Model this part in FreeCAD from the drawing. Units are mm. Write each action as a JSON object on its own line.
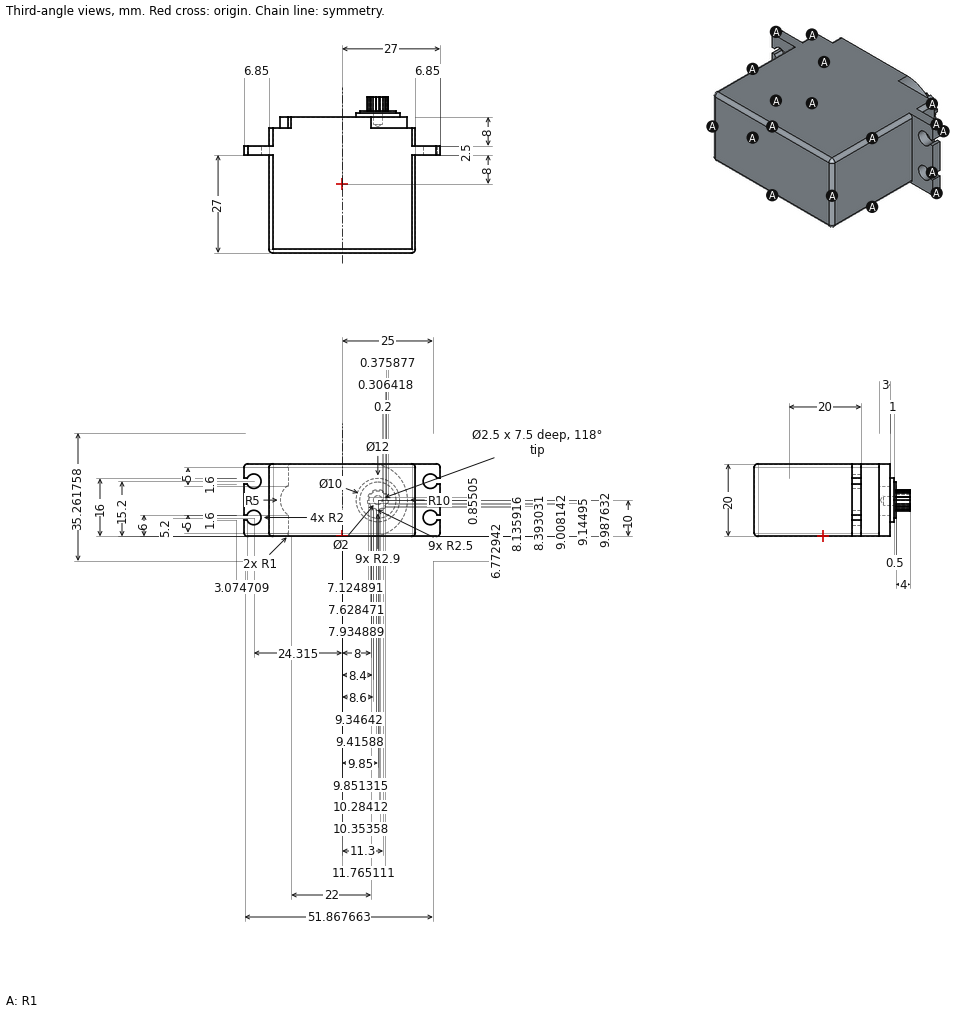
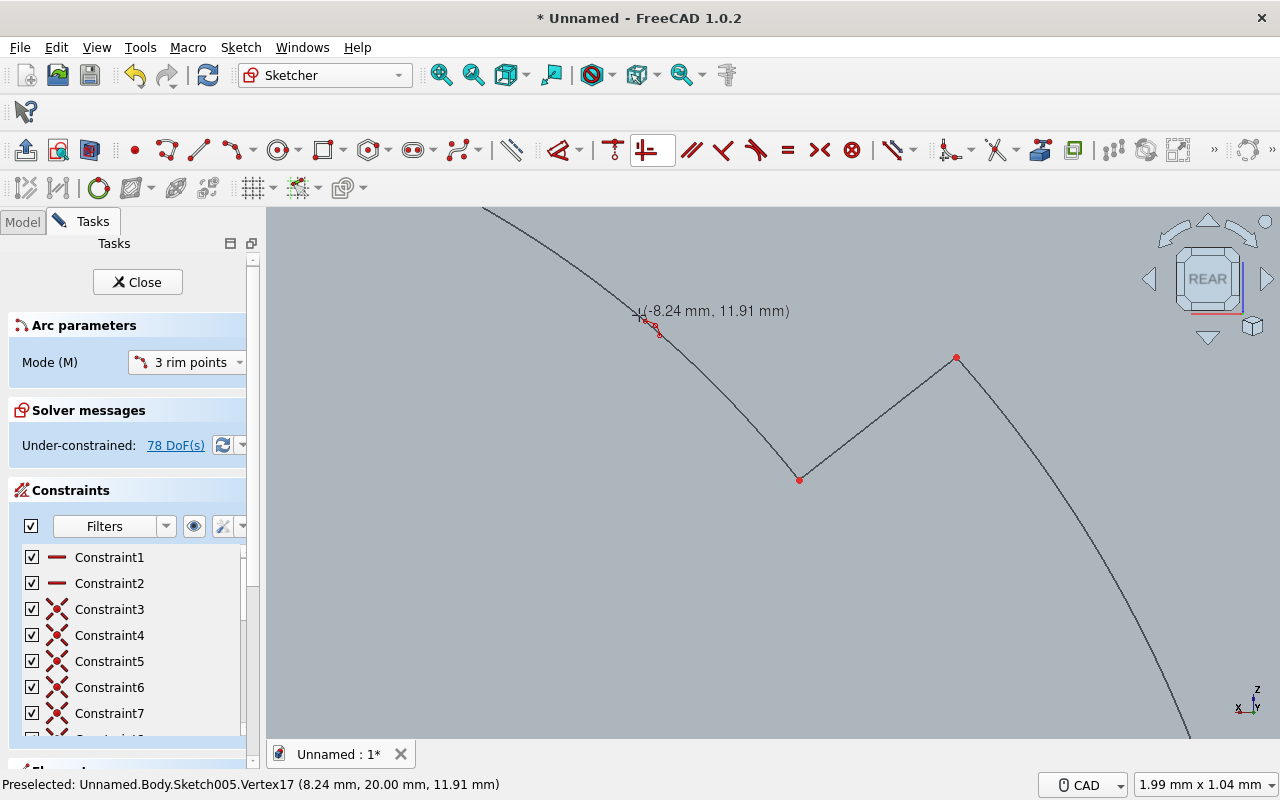
{"action": "scroll", "coordinate": [658, 335], "scroll_direction": "down", "scroll_amount": 15}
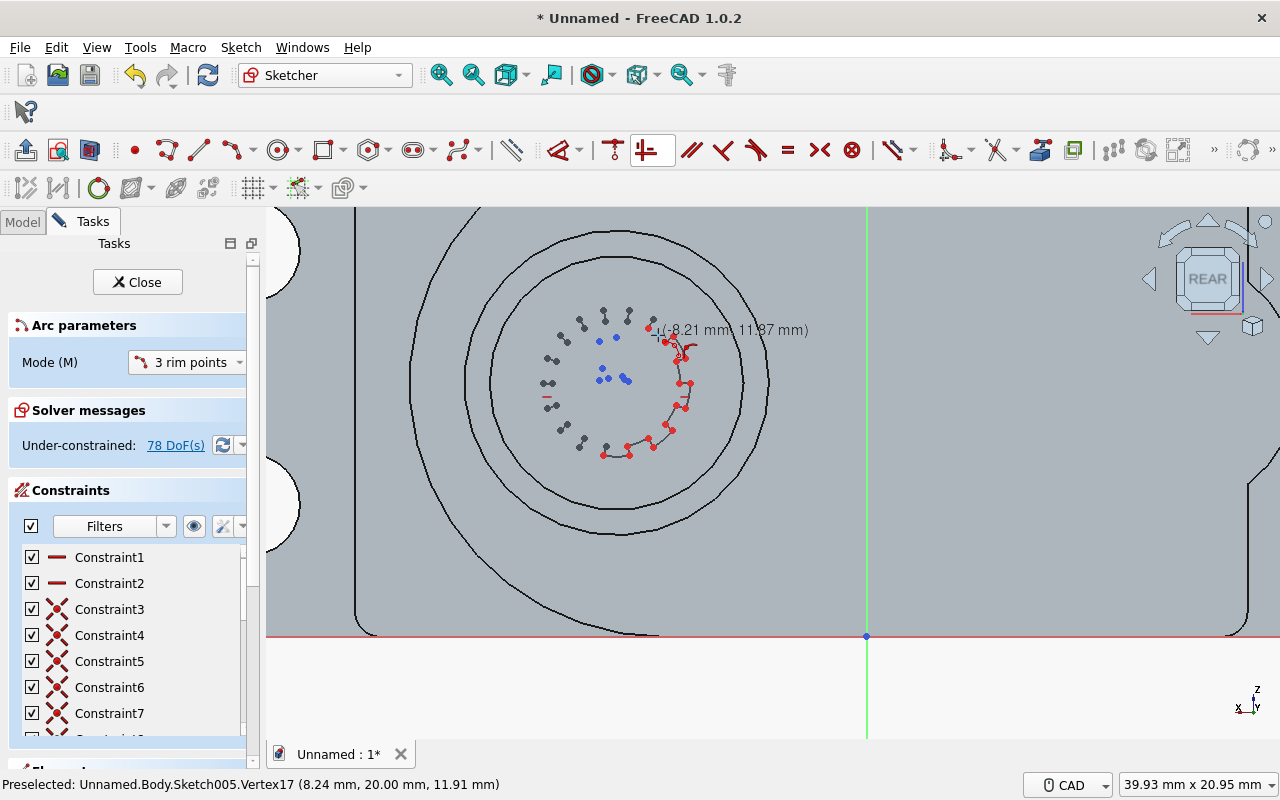
{"action": "scroll", "coordinate": [653, 319], "scroll_direction": "up", "scroll_amount": 6}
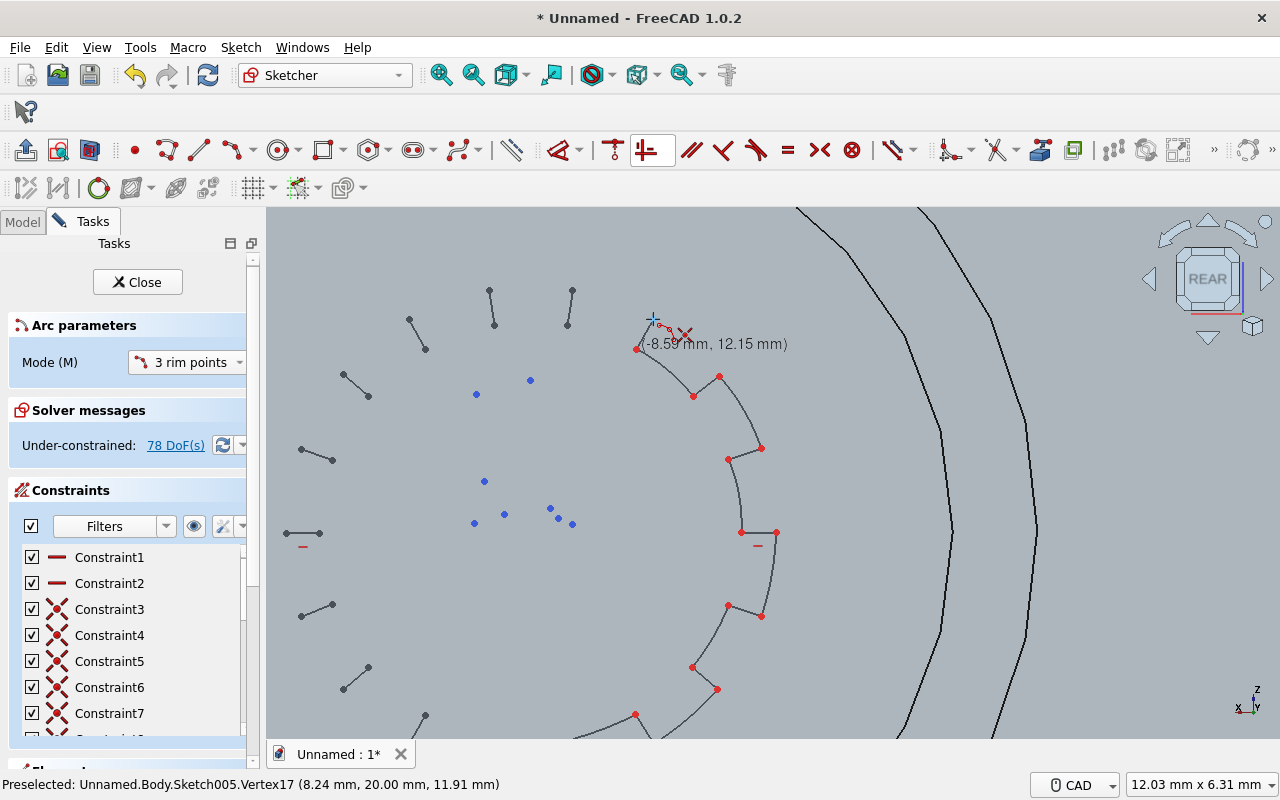
{"action": "left_click", "coordinate": [653, 320]}
{"action": "left_click", "coordinate": [573, 291]}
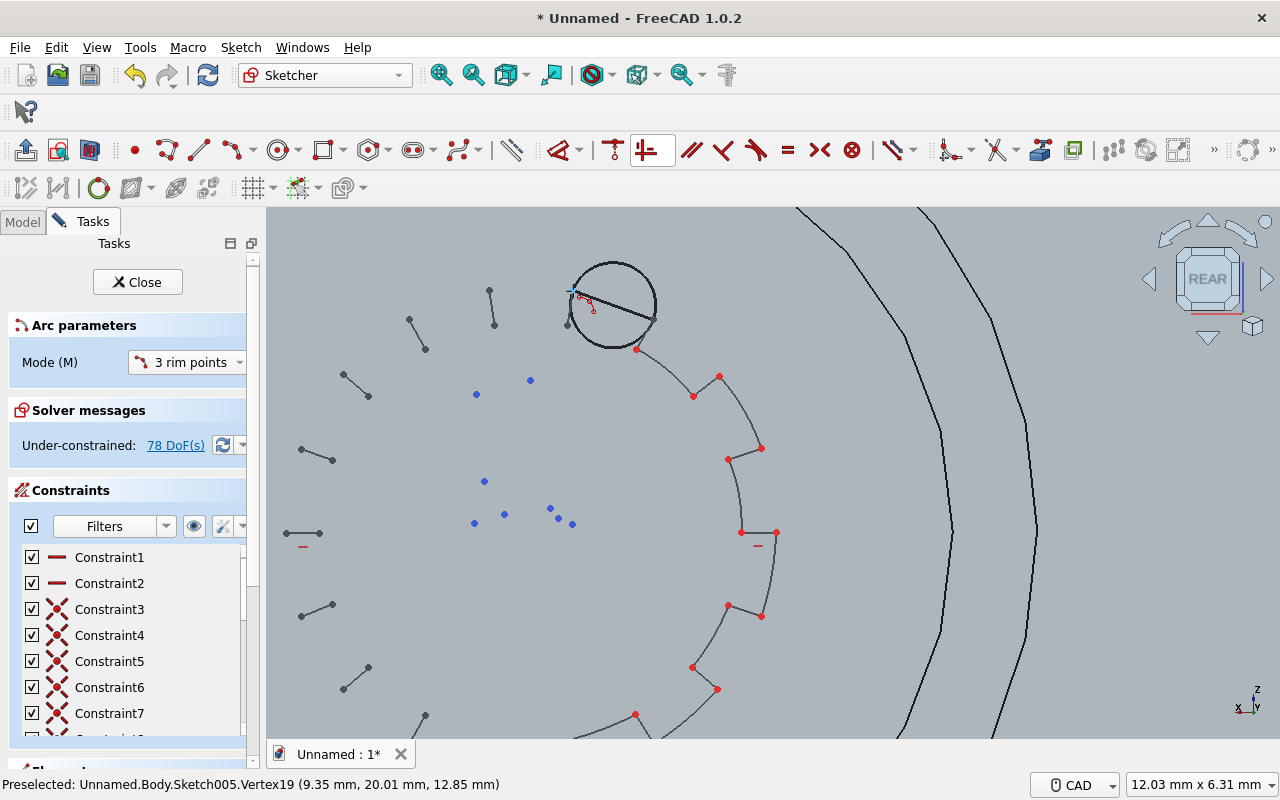
{"action": "scroll", "coordinate": [615, 301], "scroll_direction": "up", "scroll_amount": 8}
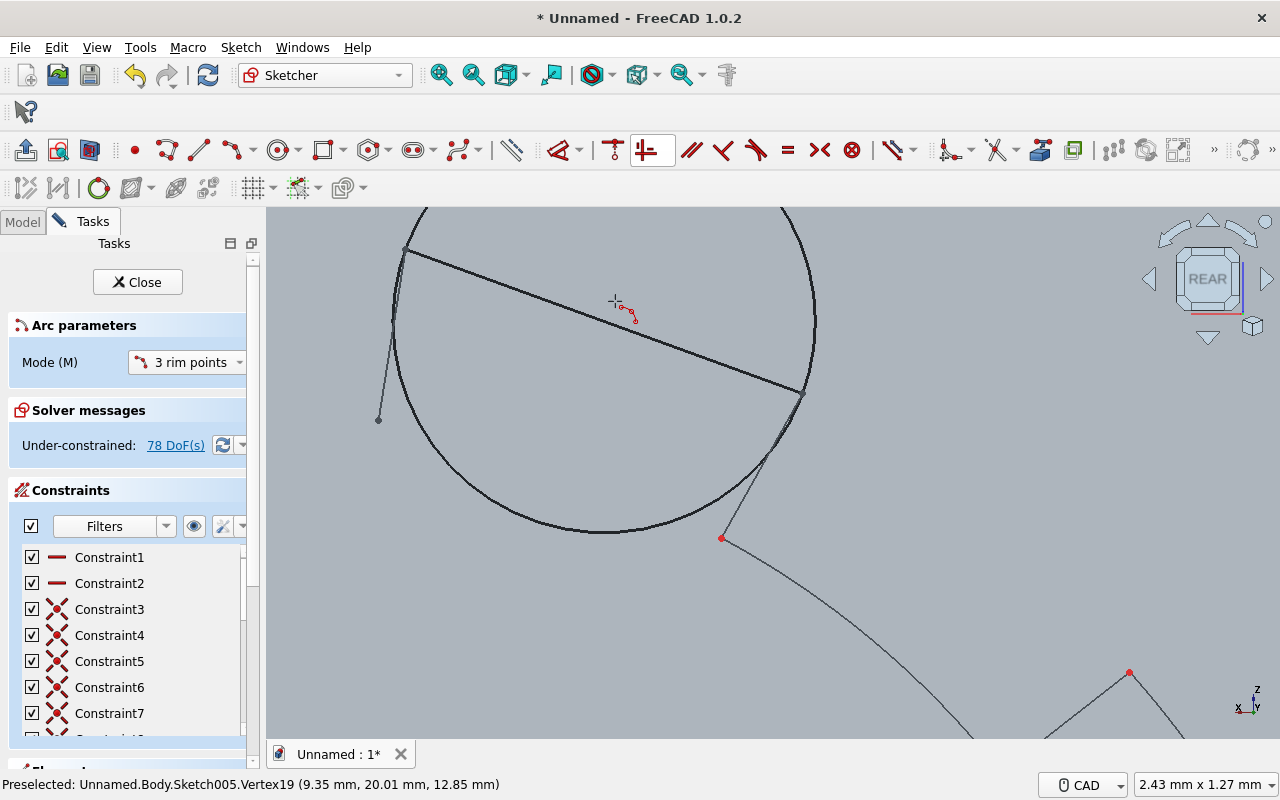
{"action": "left_click", "coordinate": [613, 299]}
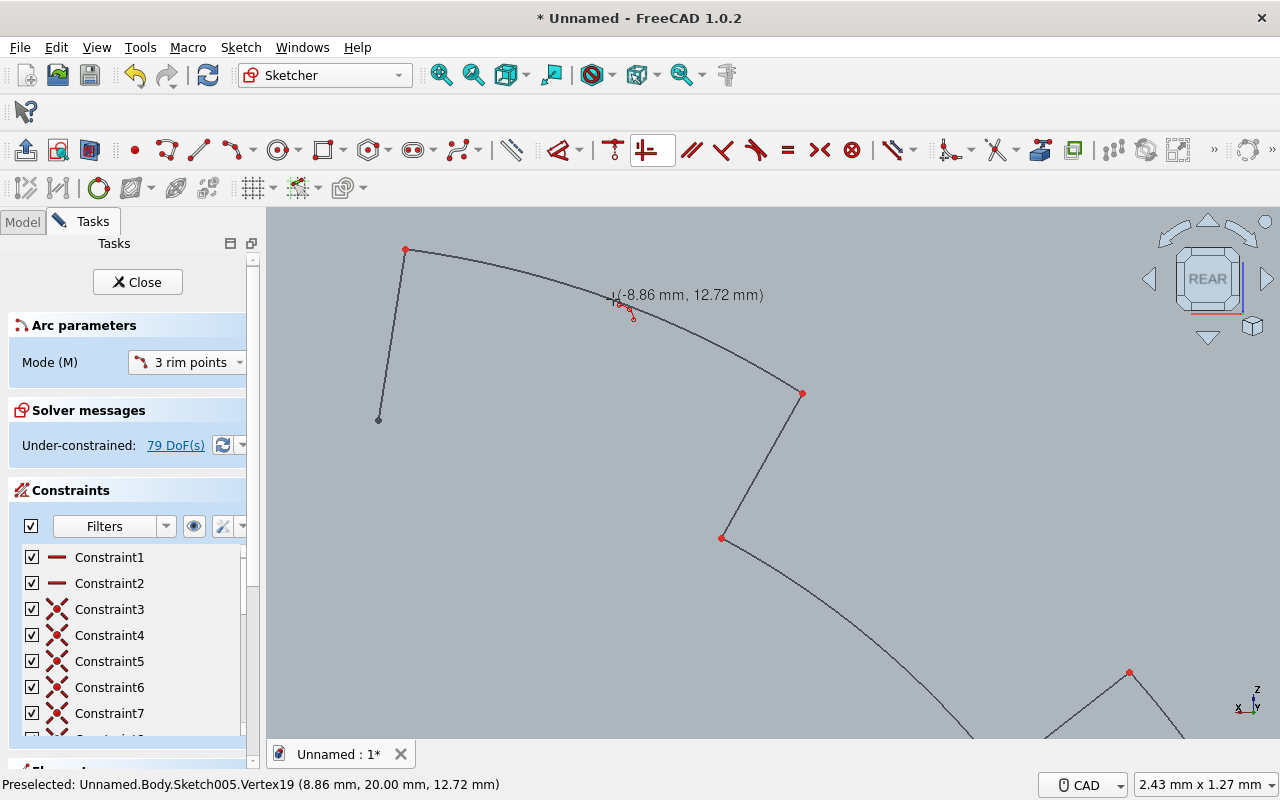
{"action": "scroll", "coordinate": [643, 314], "scroll_direction": "down", "scroll_amount": 14}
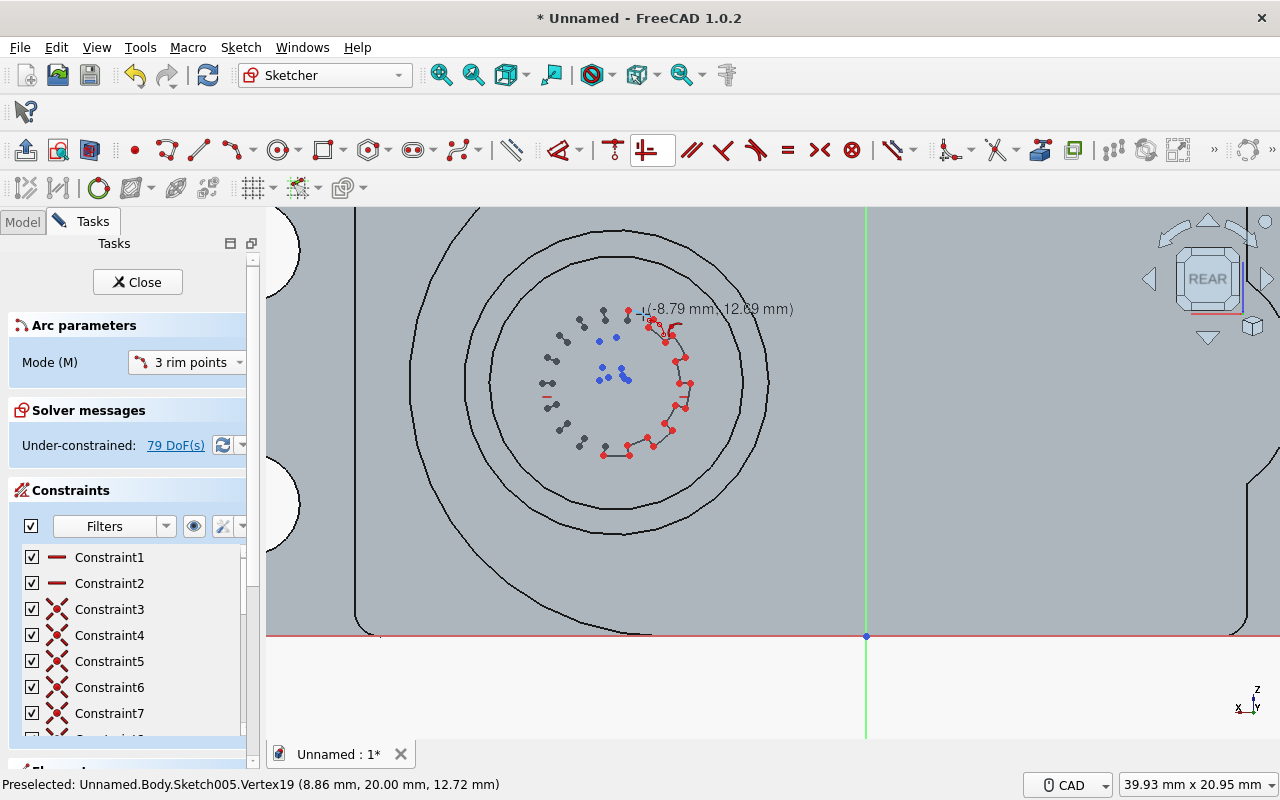
{"action": "scroll", "coordinate": [627, 320], "scroll_direction": "up", "scroll_amount": 6}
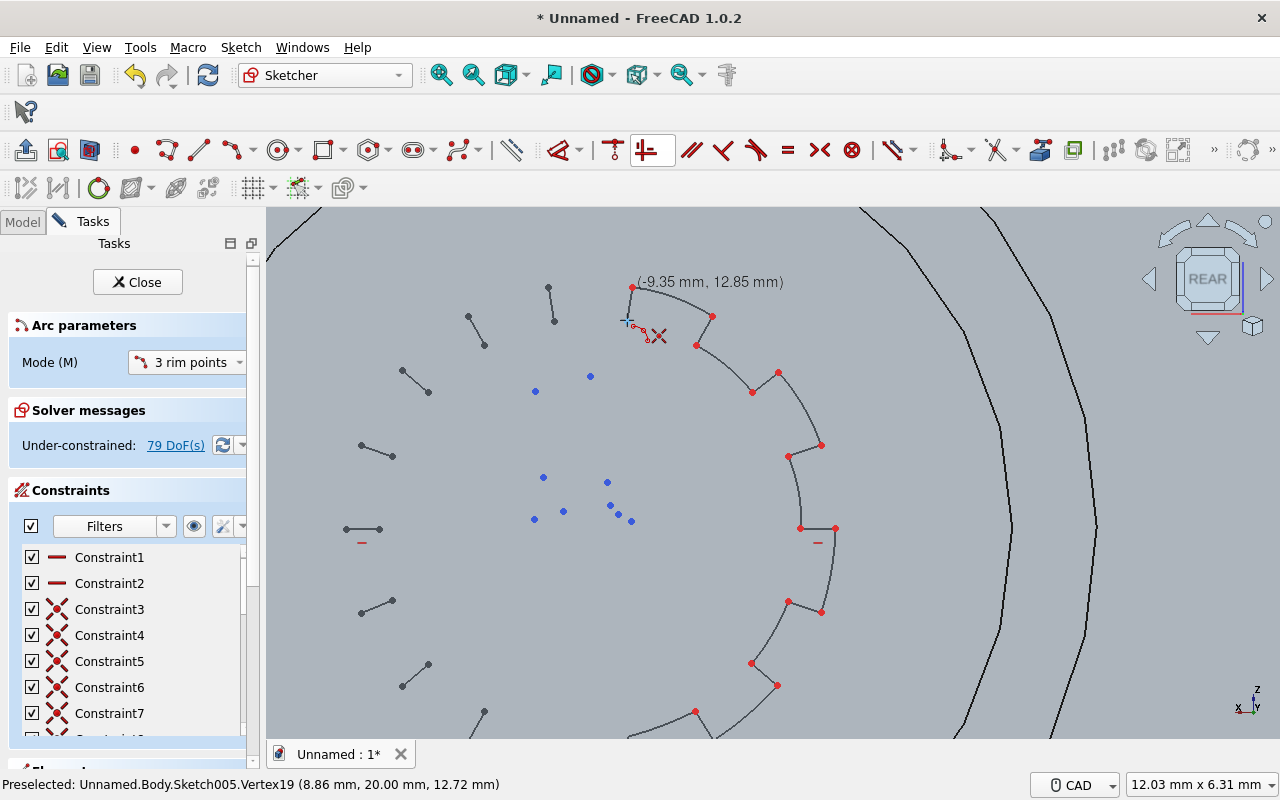
{"action": "left_click", "coordinate": [627, 322]}
{"action": "left_click", "coordinate": [554, 322]}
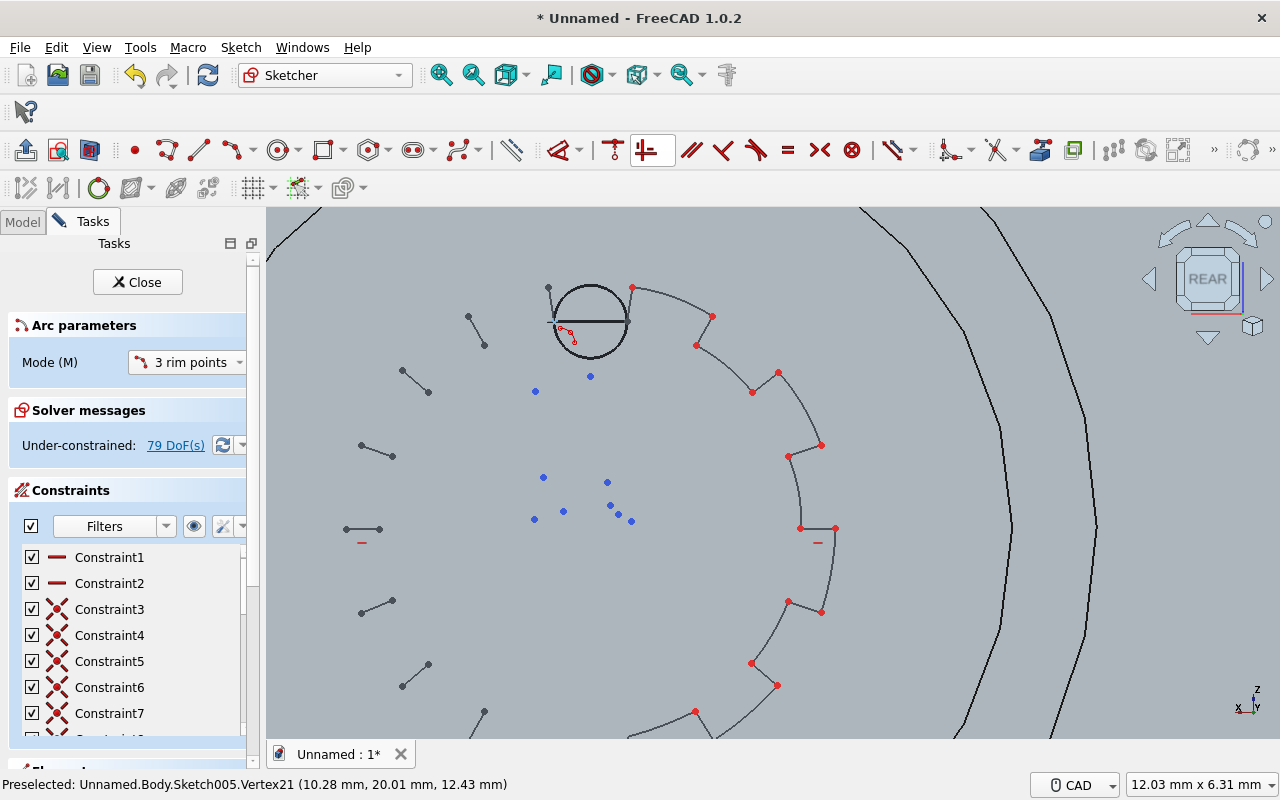
{"action": "scroll", "coordinate": [591, 316], "scroll_direction": "up", "scroll_amount": 9}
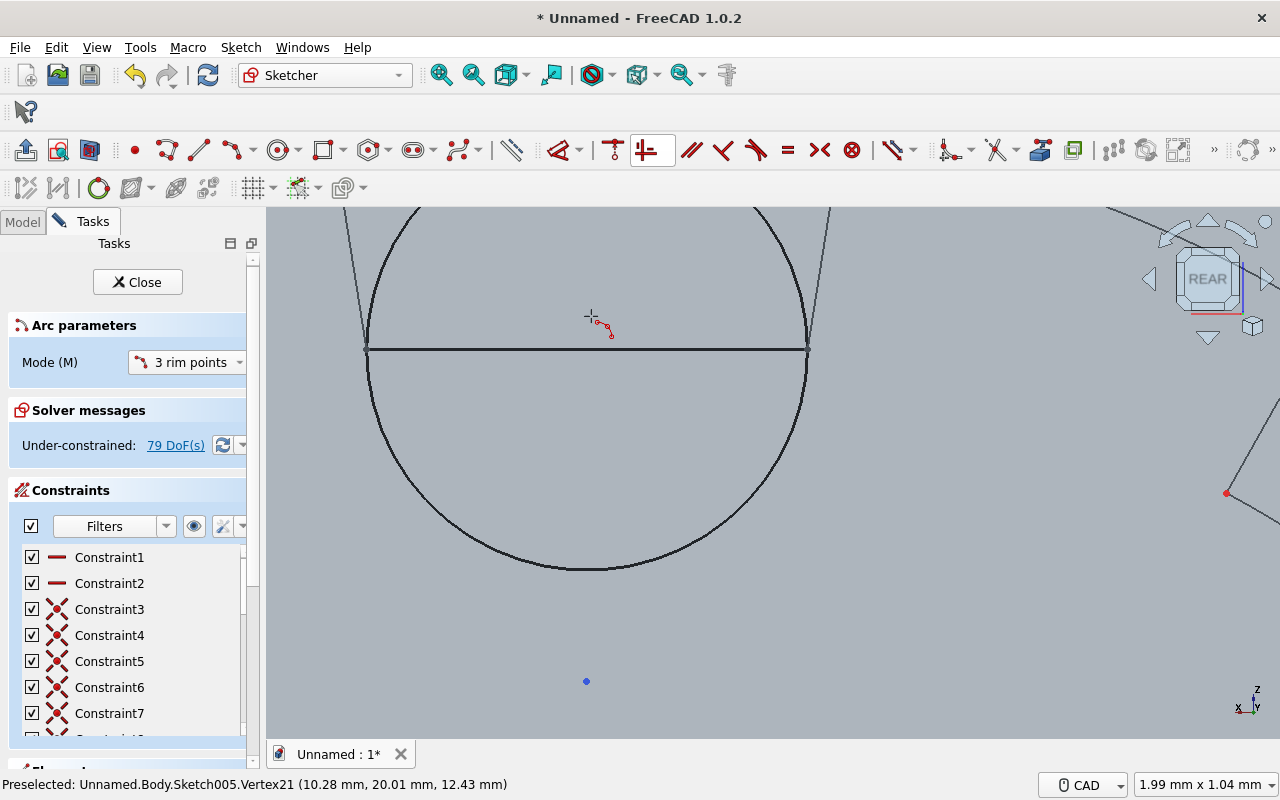
{"action": "left_click", "coordinate": [588, 316]}